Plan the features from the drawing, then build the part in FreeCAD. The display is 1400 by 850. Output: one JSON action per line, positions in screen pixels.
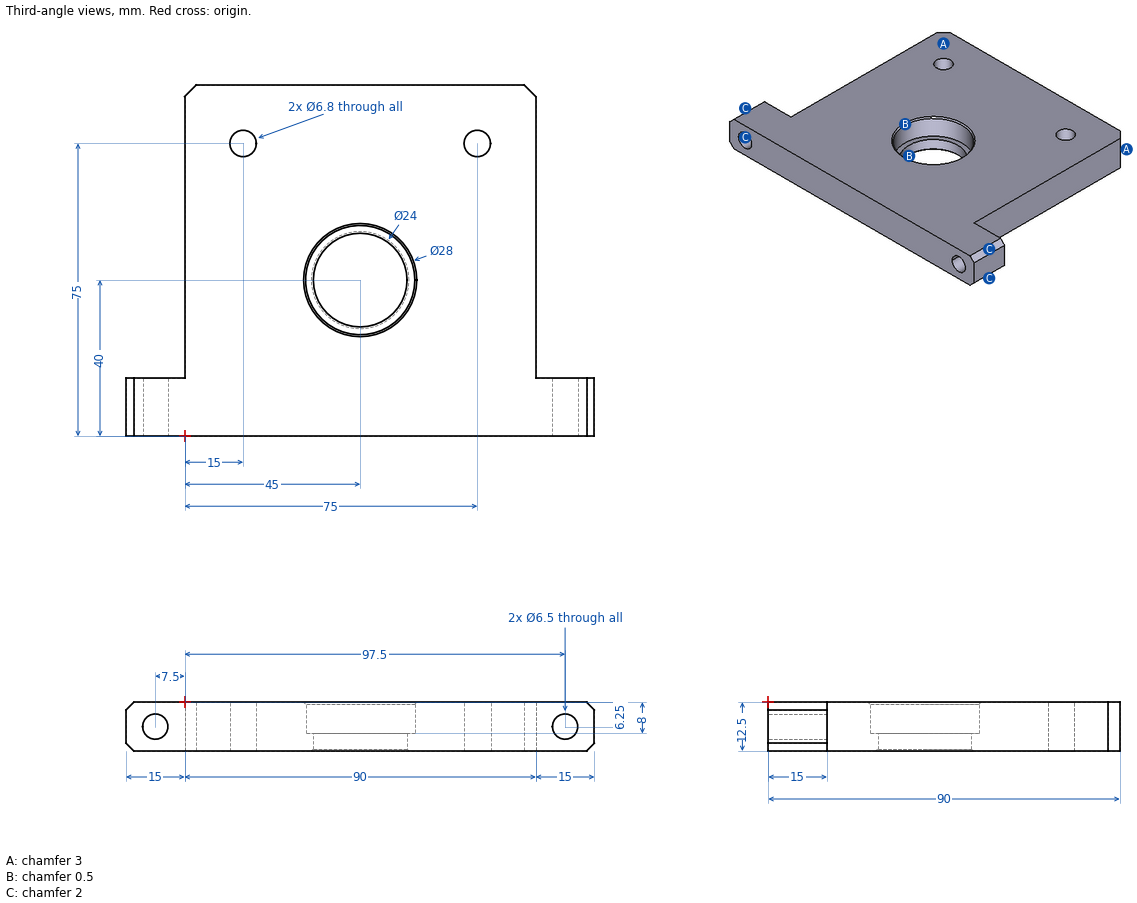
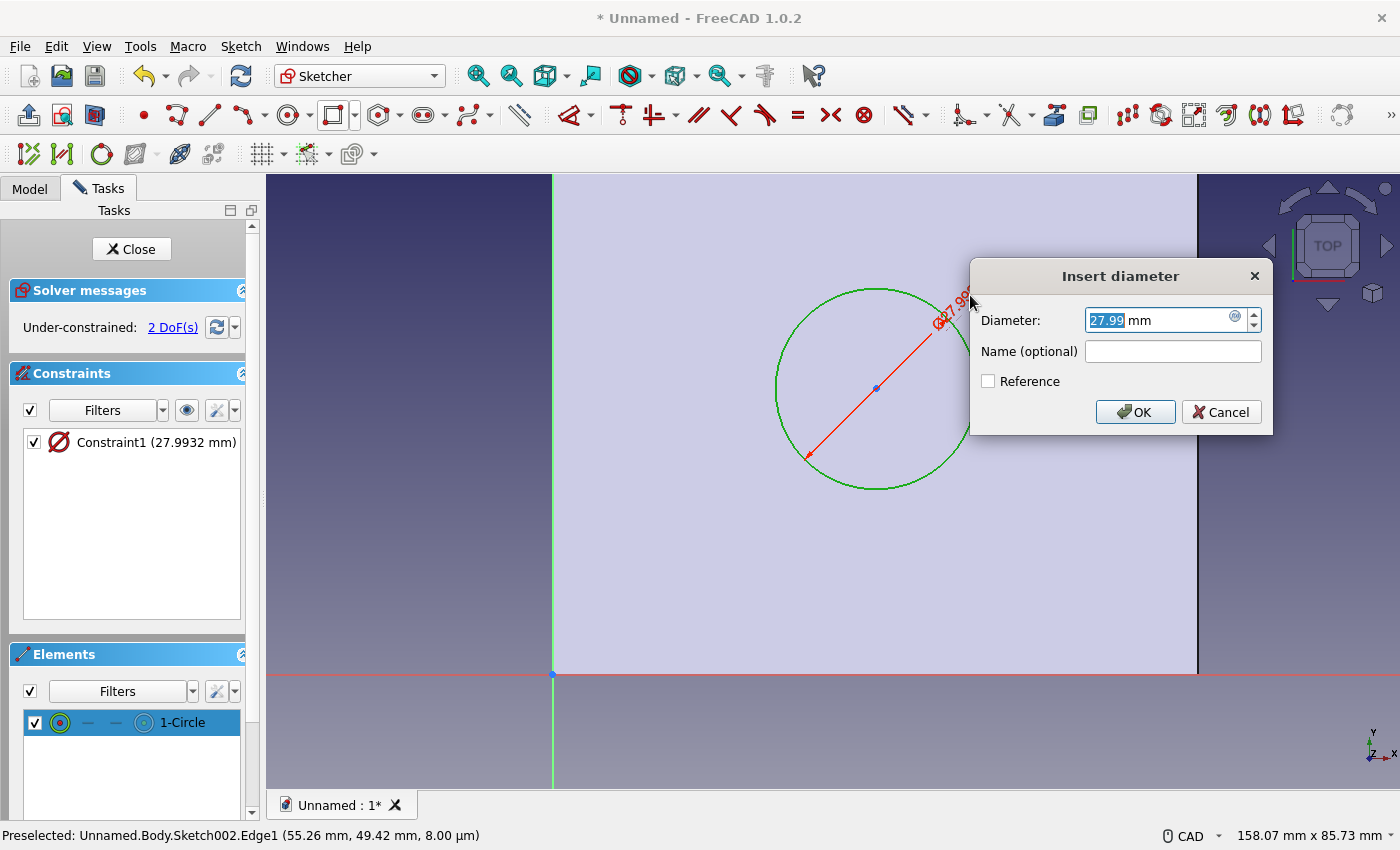
{"action": "type", "text": "28"}
{"action": "key", "text": "Return"}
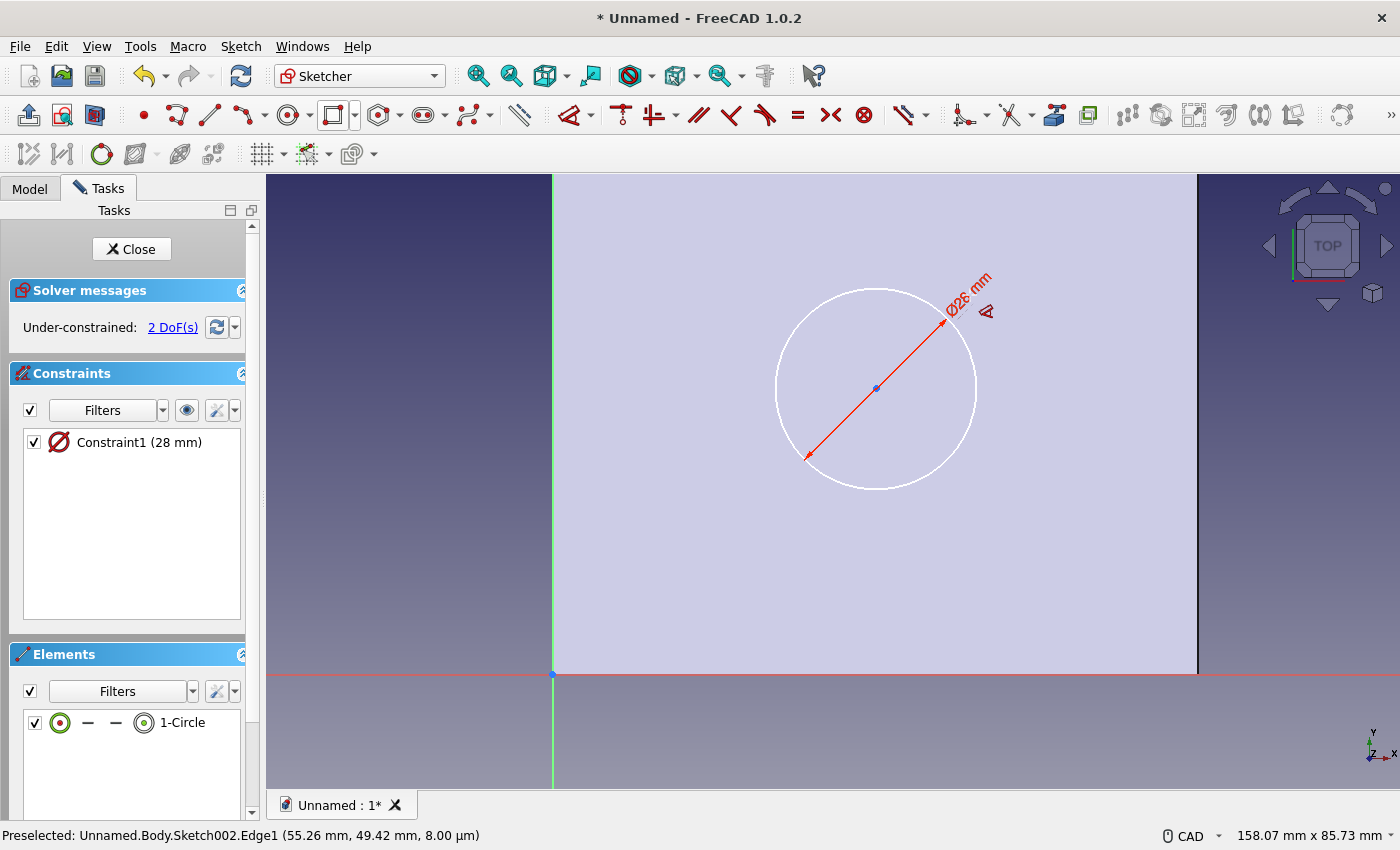
{"action": "left_click", "coordinate": [876, 389]}
{"action": "left_click", "coordinate": [714, 709]}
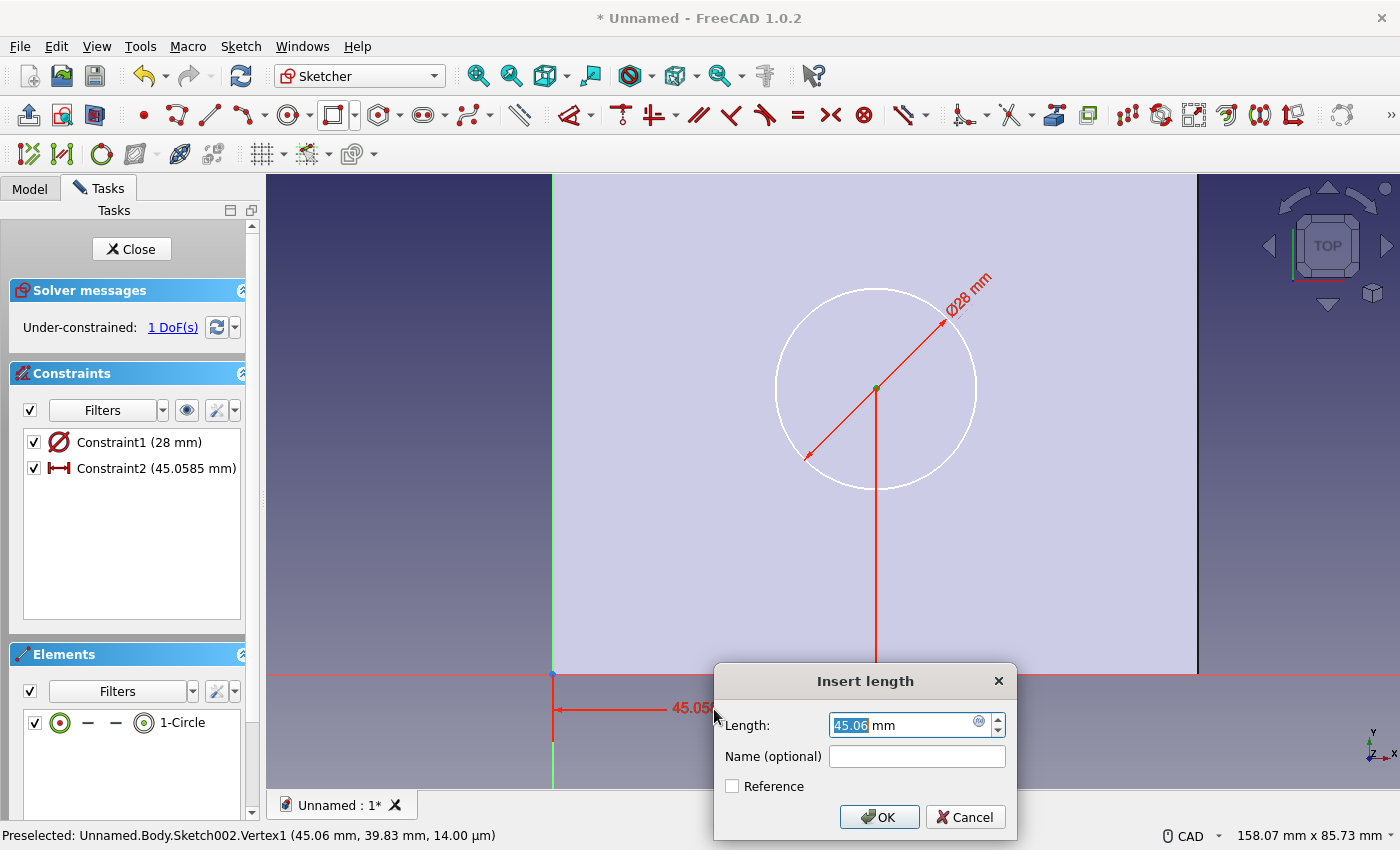
{"action": "type", "text": "45"}
{"action": "key", "text": "Return"}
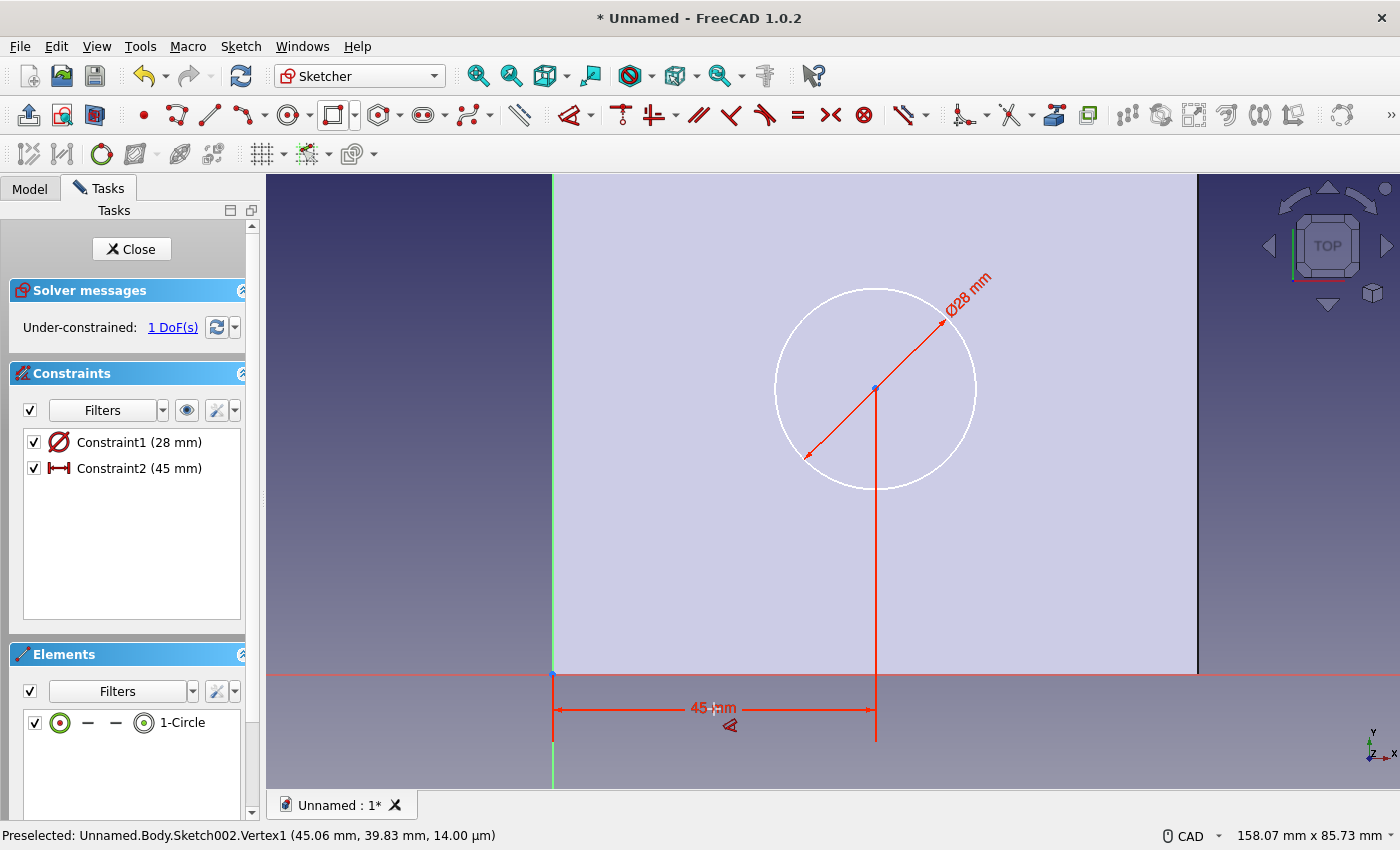
{"action": "left_click", "coordinate": [876, 389]}
{"action": "left_click", "coordinate": [519, 532]}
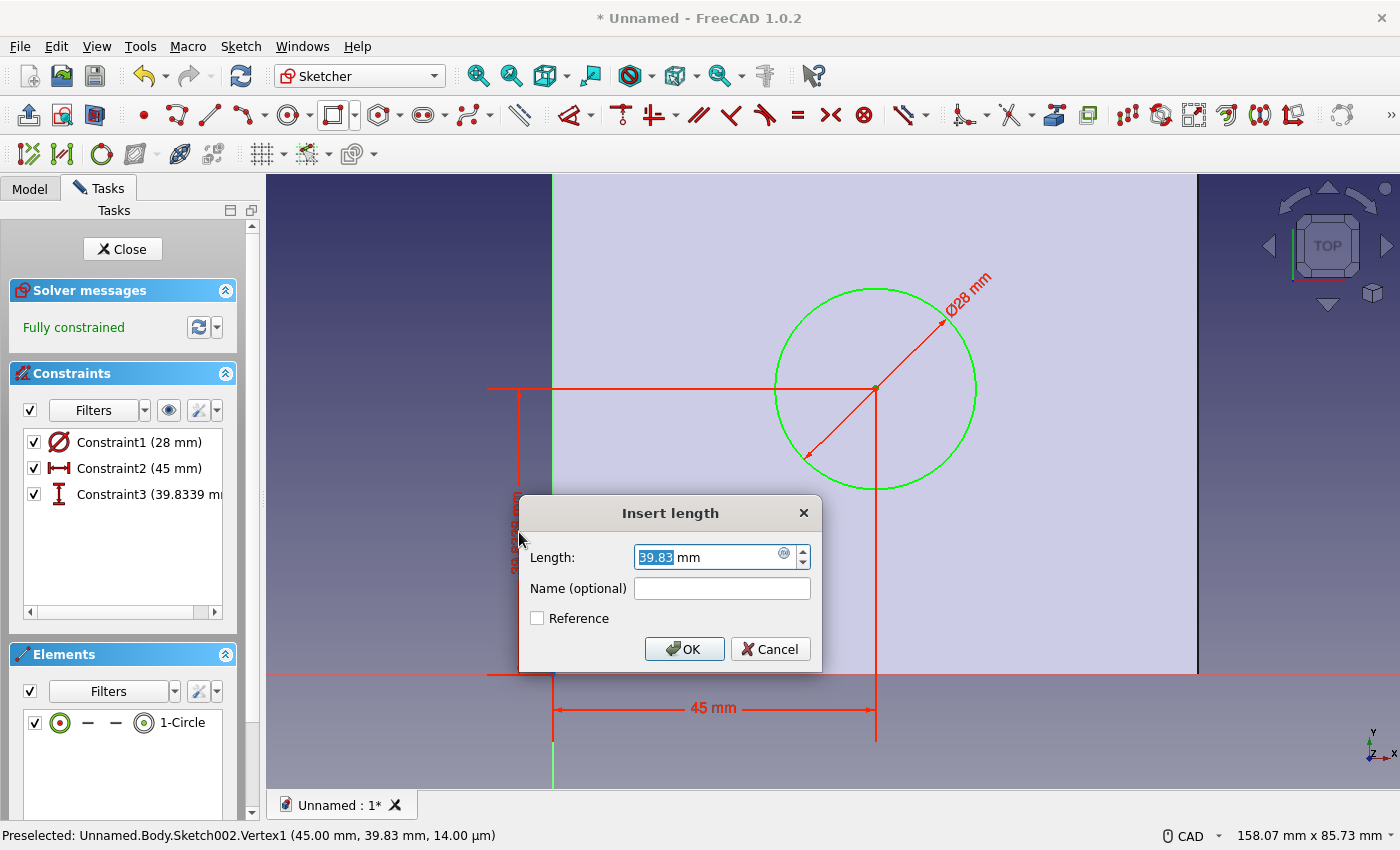
{"action": "type", "text": "40"}
{"action": "key", "text": "Return"}
{"action": "key", "text": "Escape"}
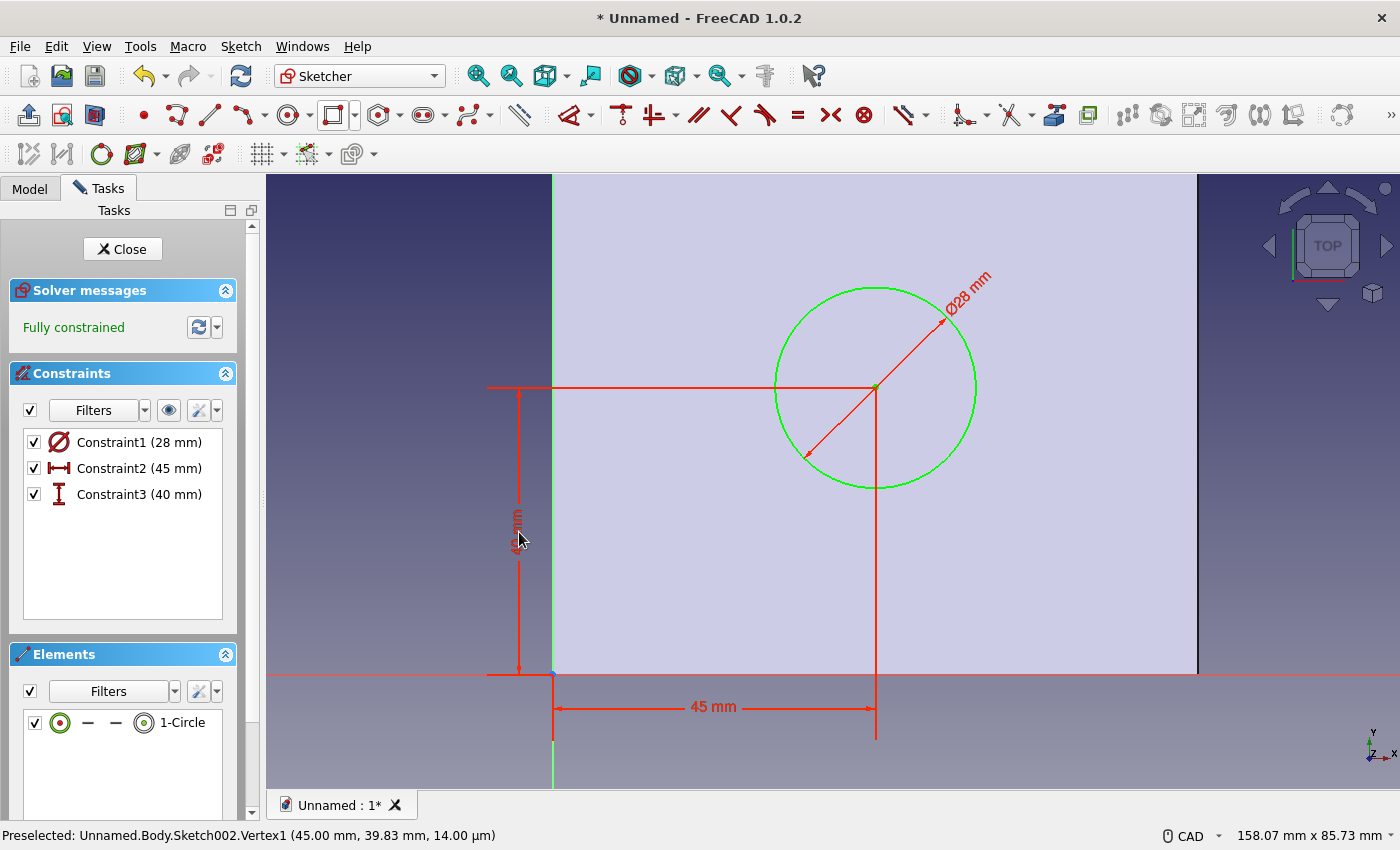
{"action": "left_click", "coordinate": [123, 249]}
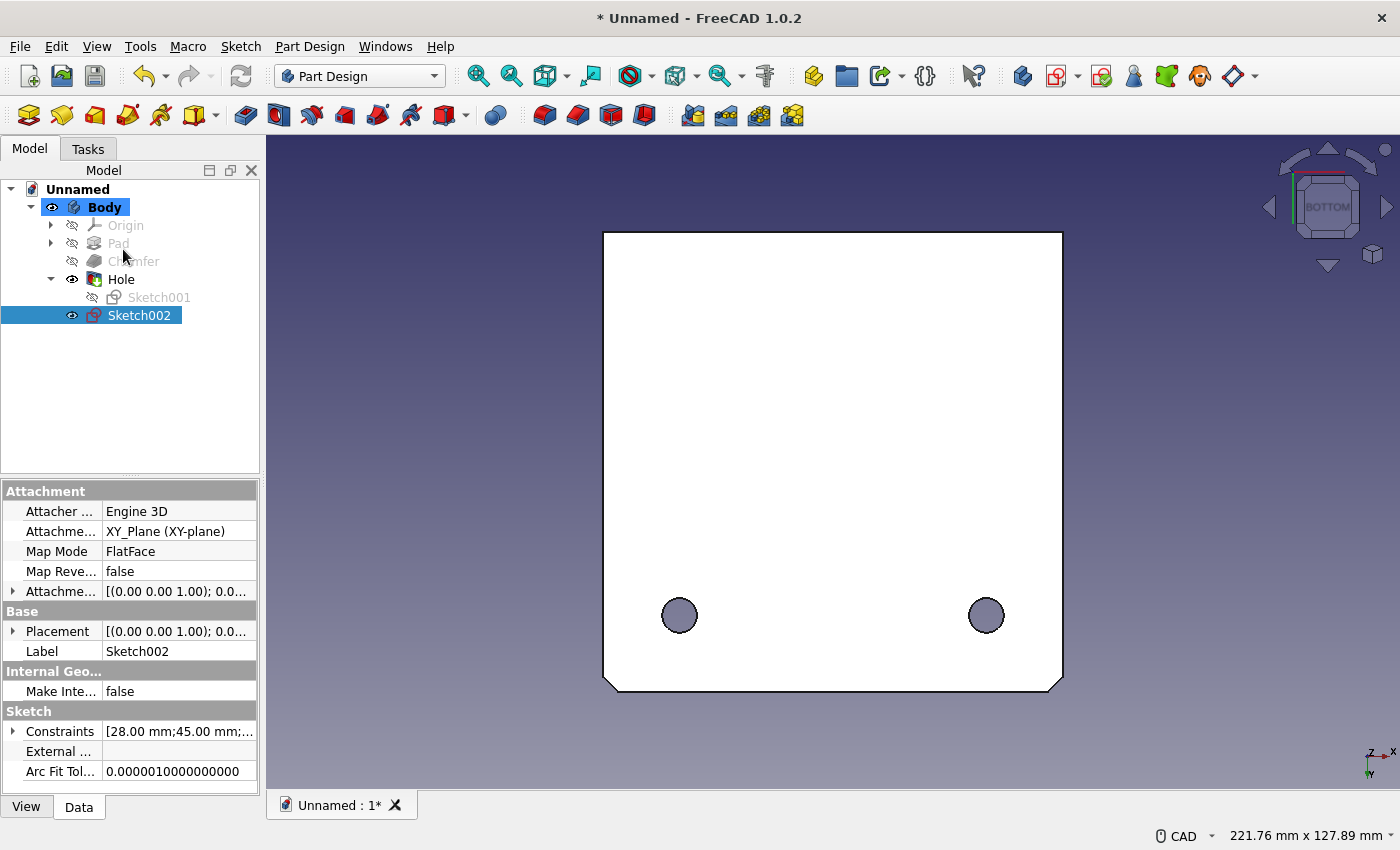
{"action": "left_click", "coordinate": [246, 116]}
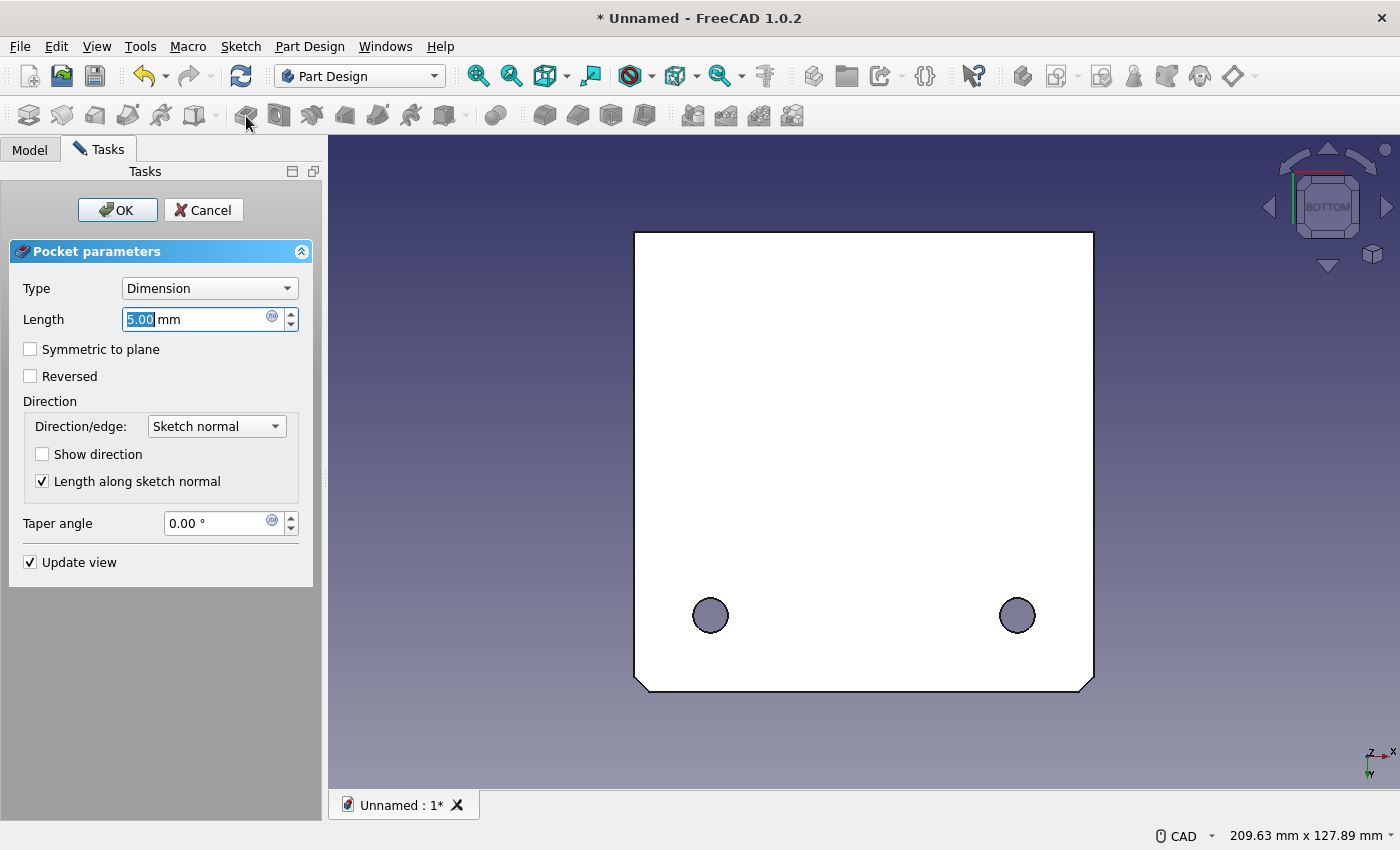
{"action": "type", "text": "8"}
{"action": "key", "text": "Tab"}